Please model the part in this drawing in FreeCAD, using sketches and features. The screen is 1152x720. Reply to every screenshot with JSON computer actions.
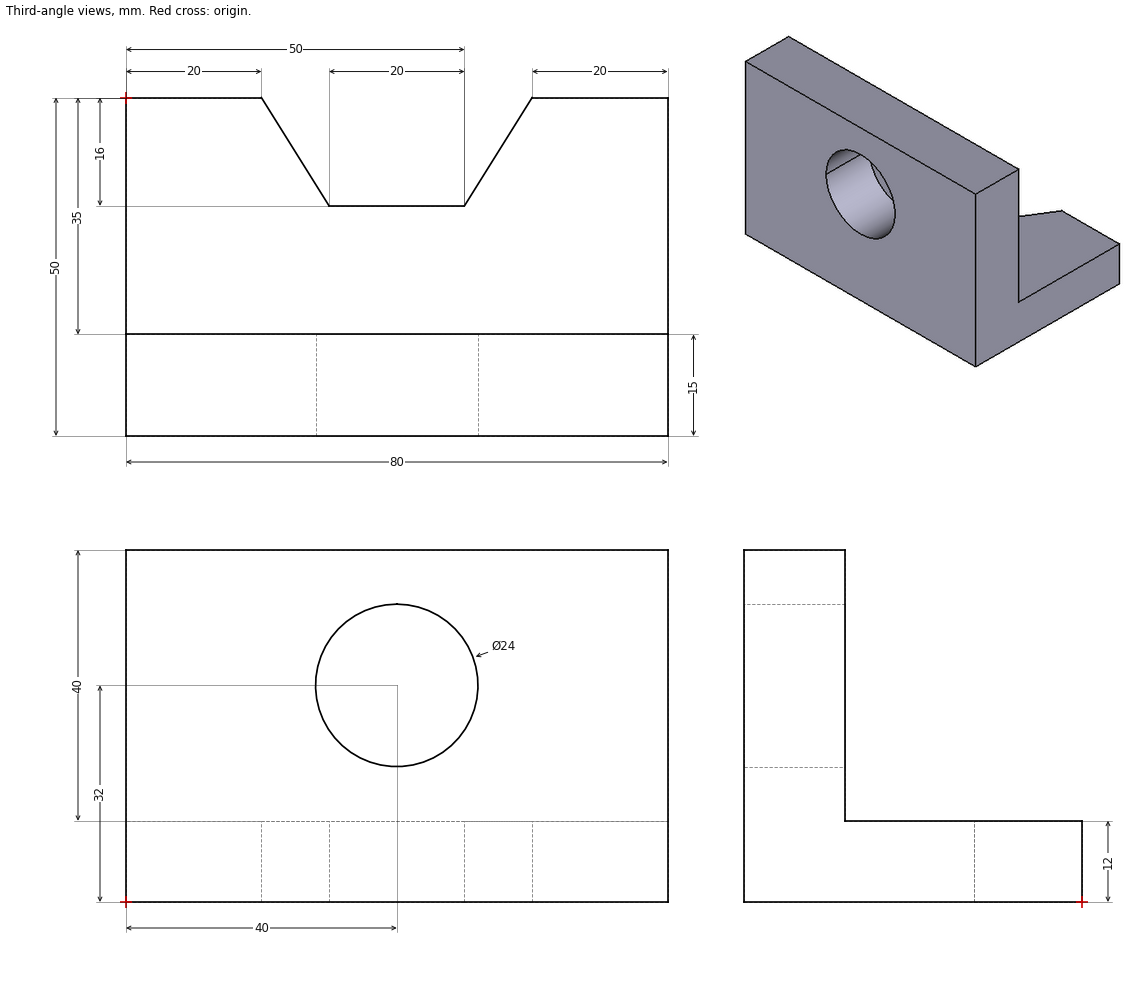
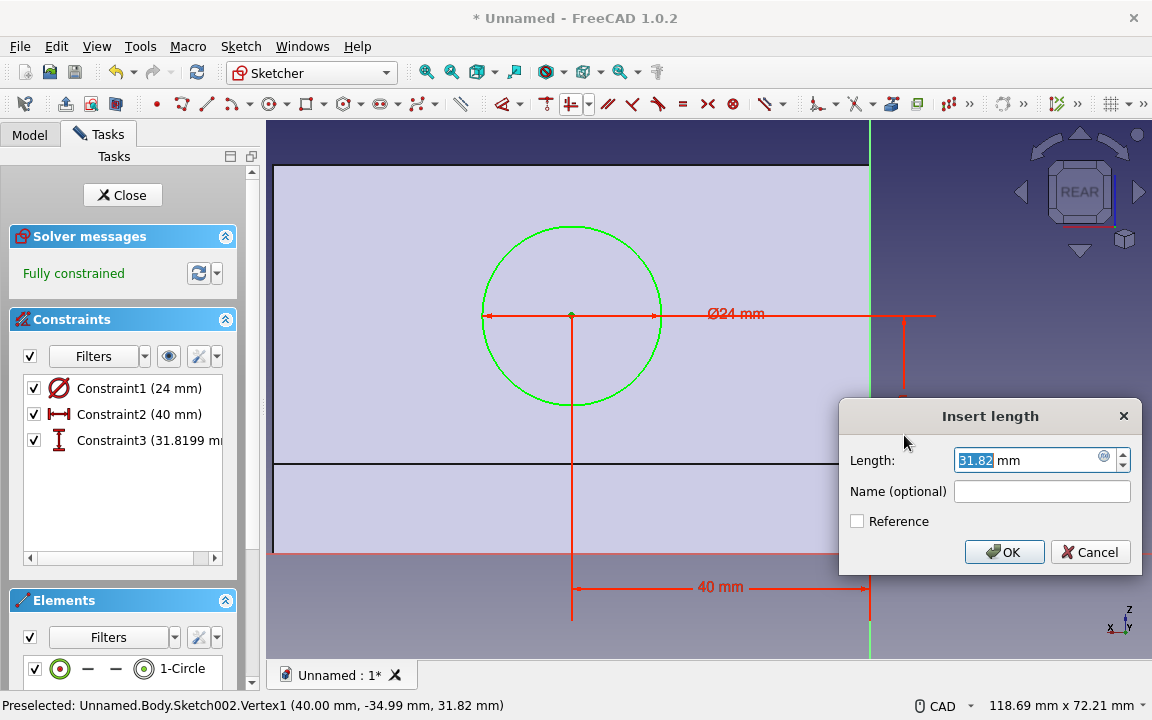
{"action": "type", "text": "32"}
{"action": "key", "text": "Return"}
{"action": "key", "text": "Escape"}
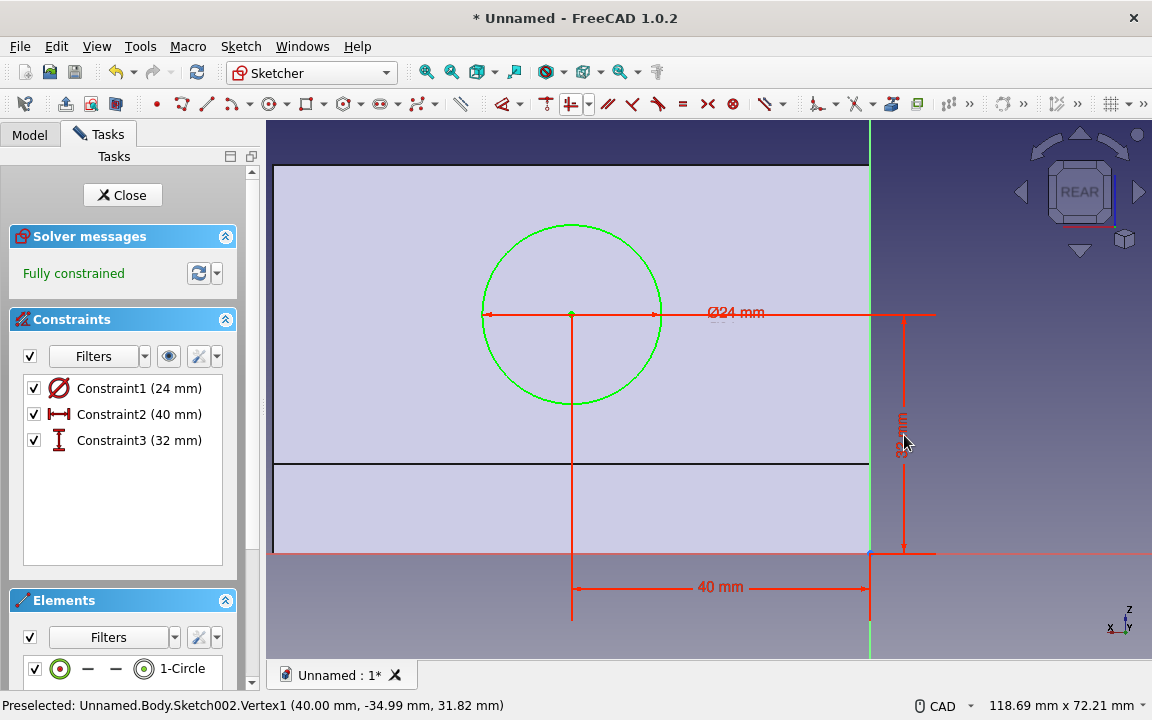
{"action": "left_click", "coordinate": [123, 195]}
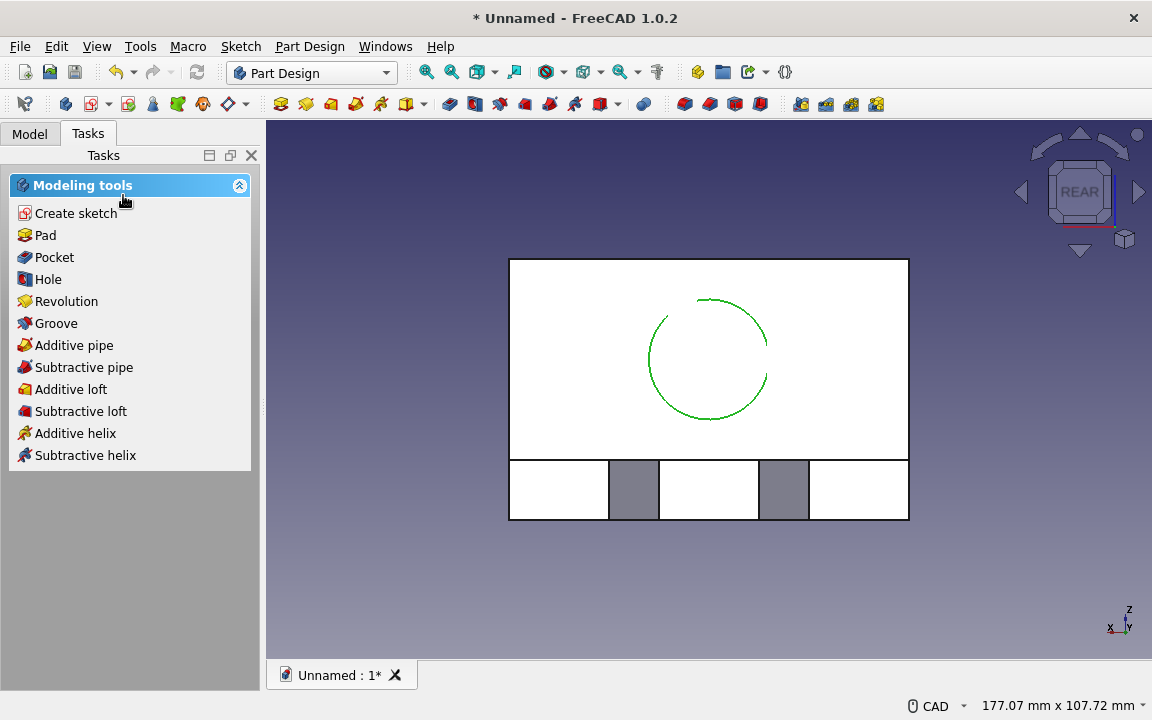
{"action": "left_click", "coordinate": [450, 104]}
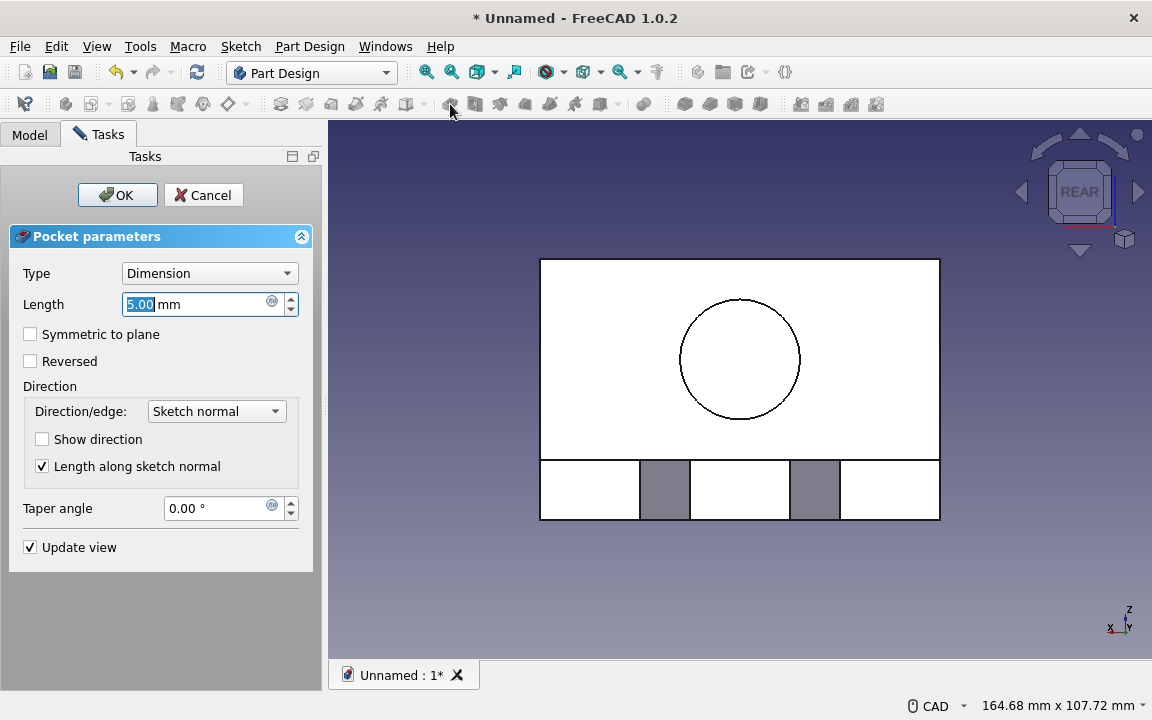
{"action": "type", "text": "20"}
{"action": "key", "text": "Tab"}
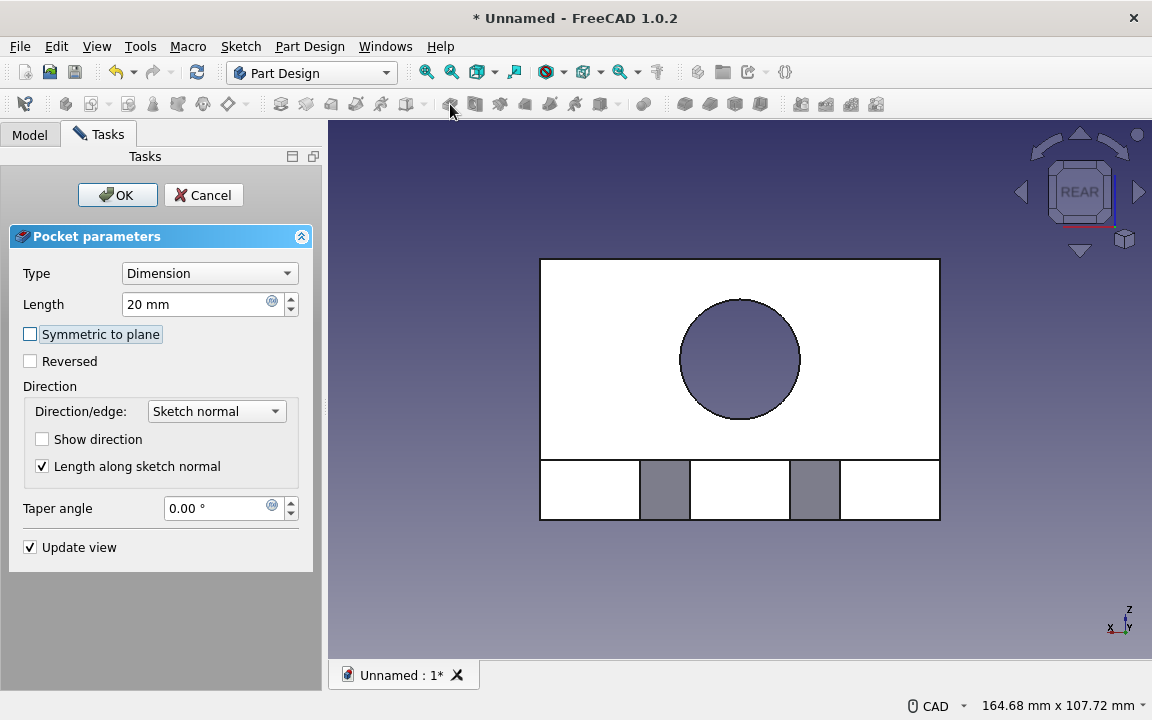
{"action": "left_click", "coordinate": [118, 195]}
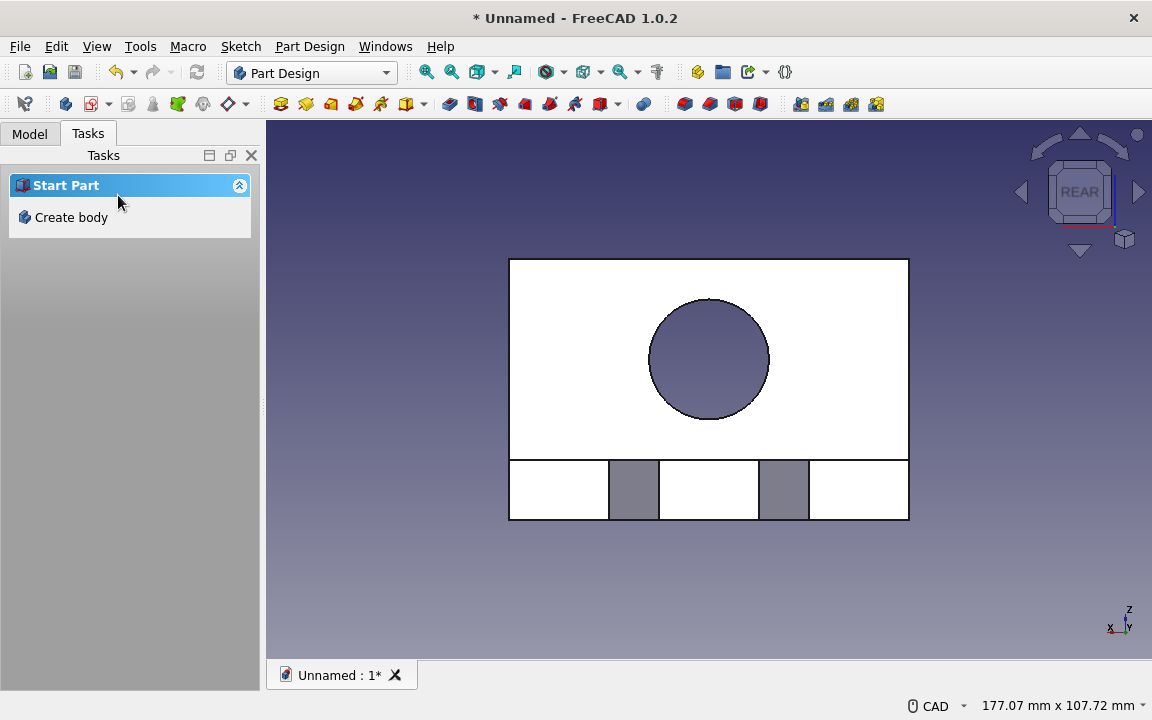
{"action": "key", "text": "0"}